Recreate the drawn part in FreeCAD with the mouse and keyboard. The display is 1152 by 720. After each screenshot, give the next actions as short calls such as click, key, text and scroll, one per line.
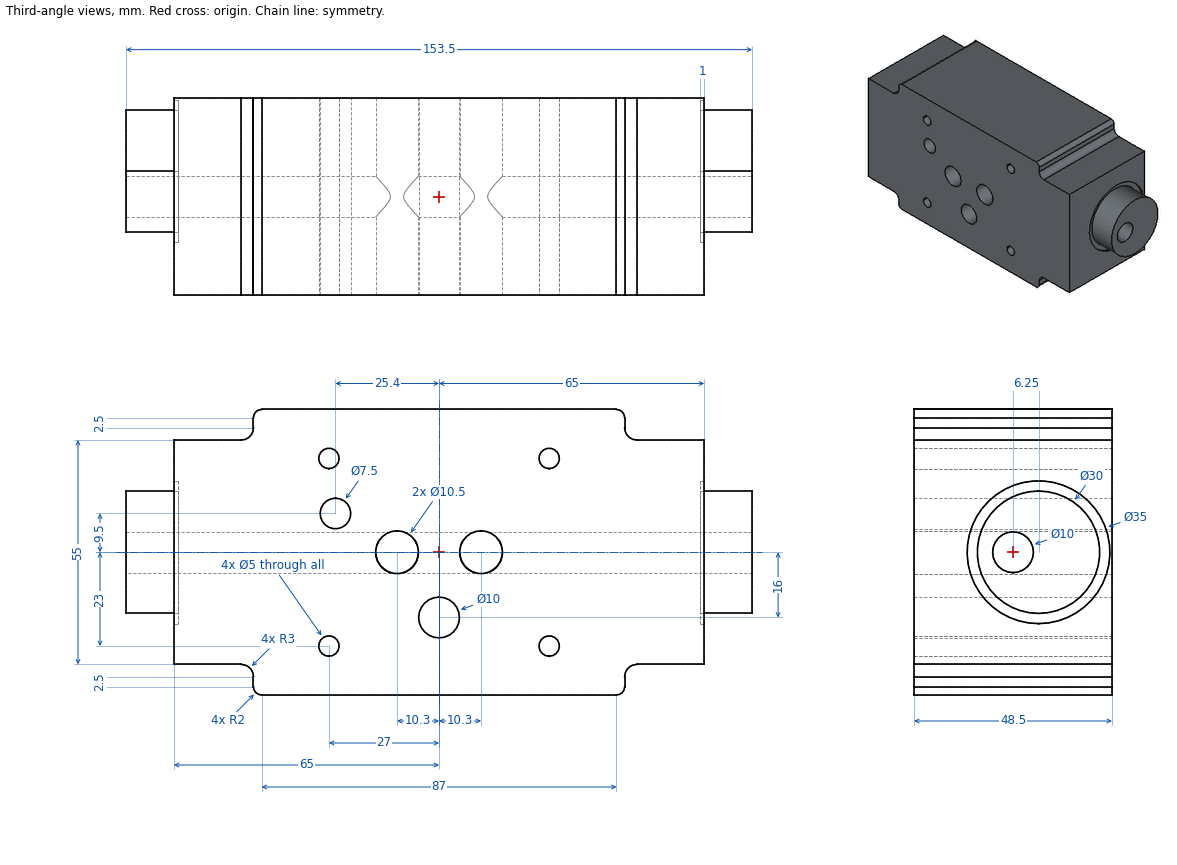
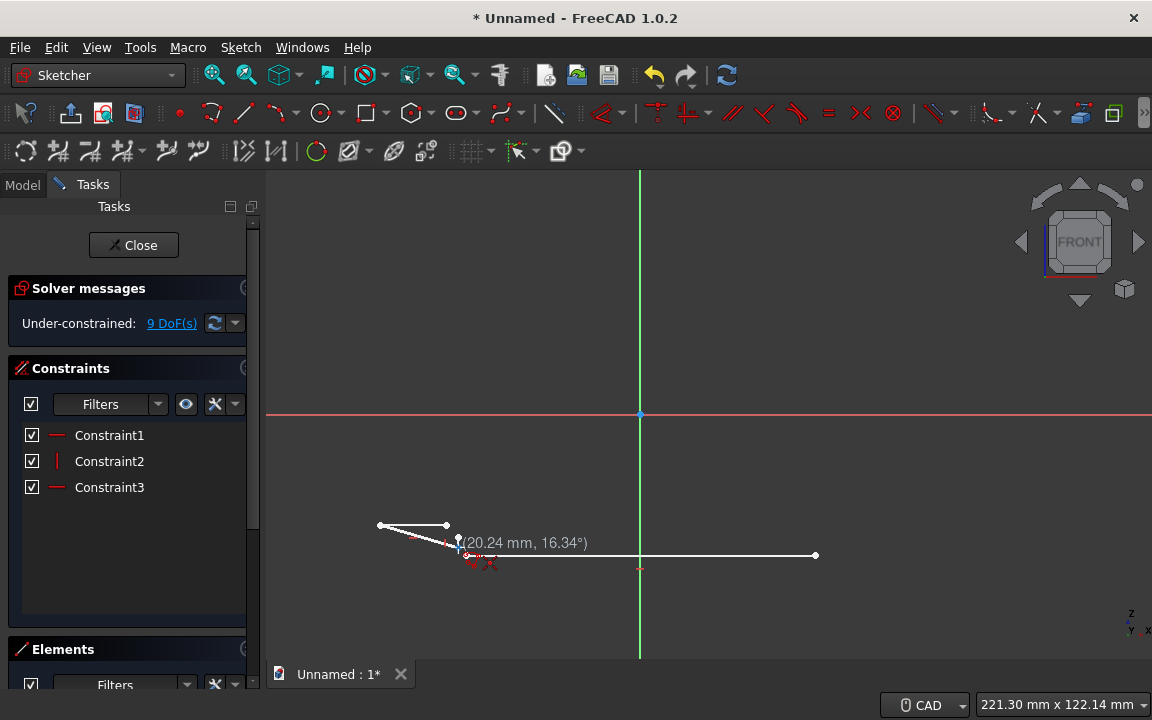
click(380, 305)
click(446, 305)
right_click(446, 305)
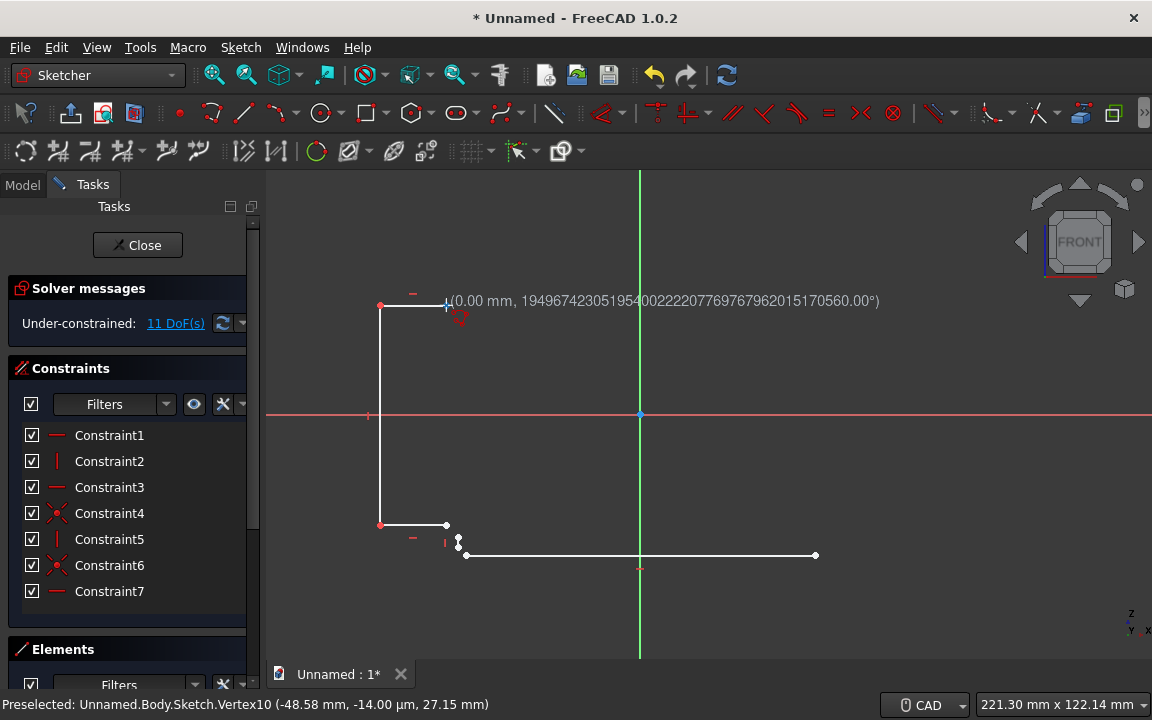
click(244, 114)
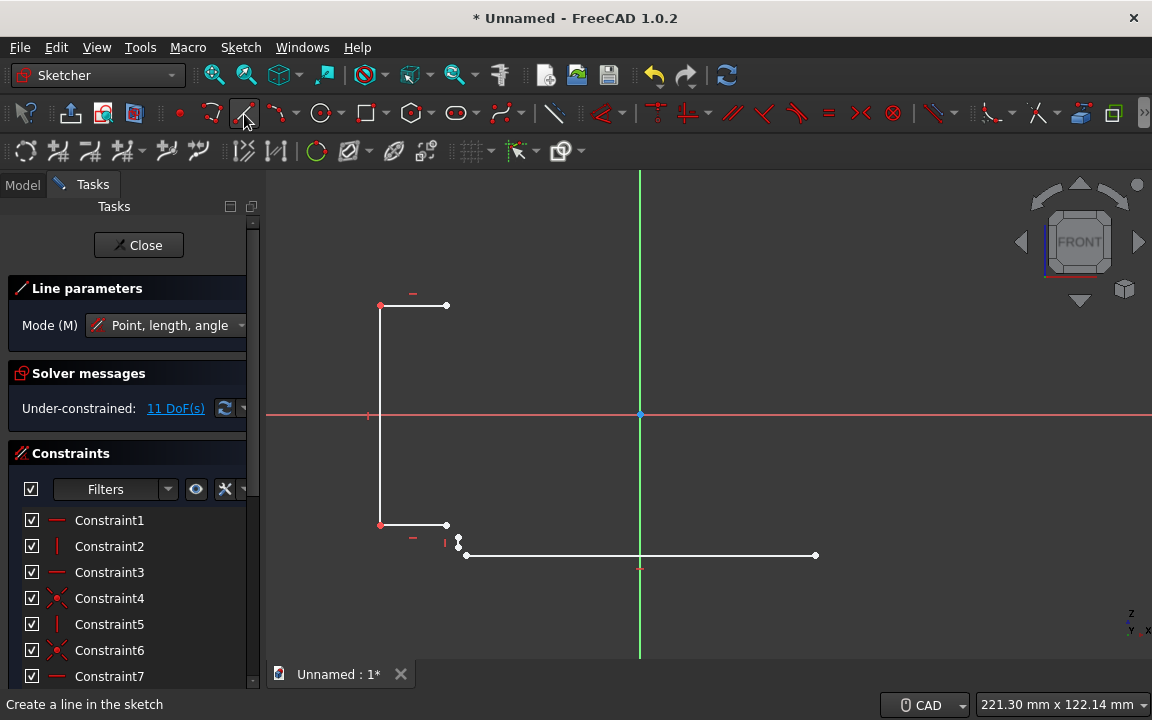
click(458, 293)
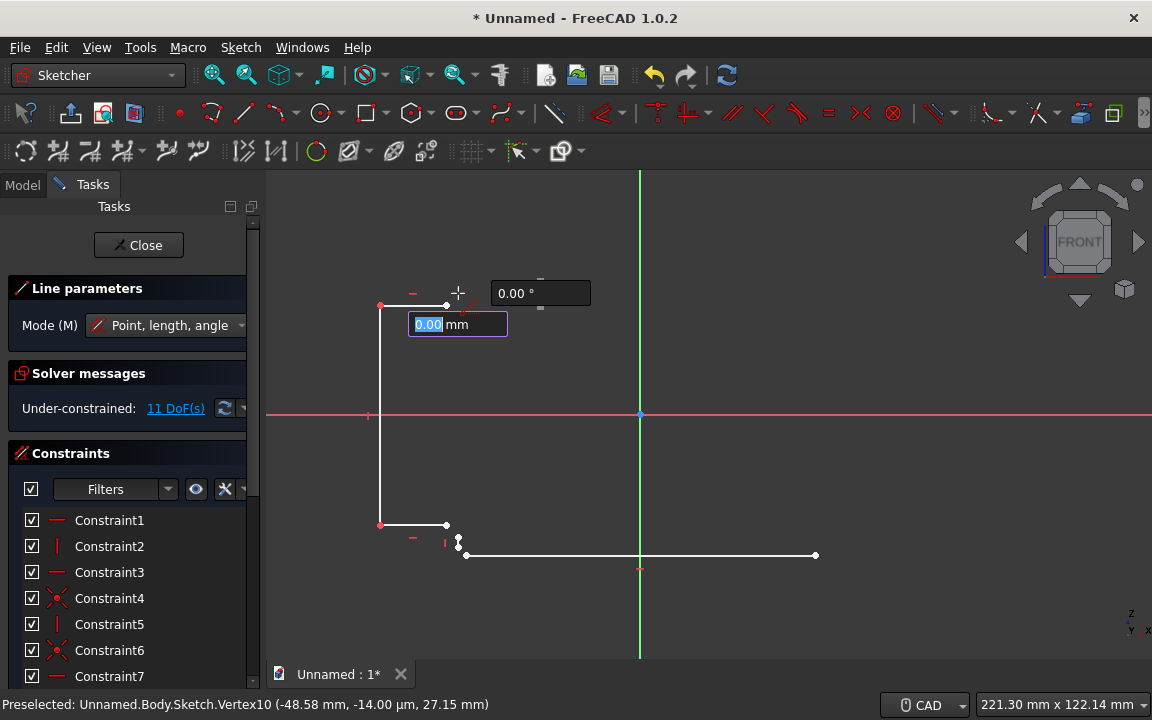
scroll(458, 283, up, 3)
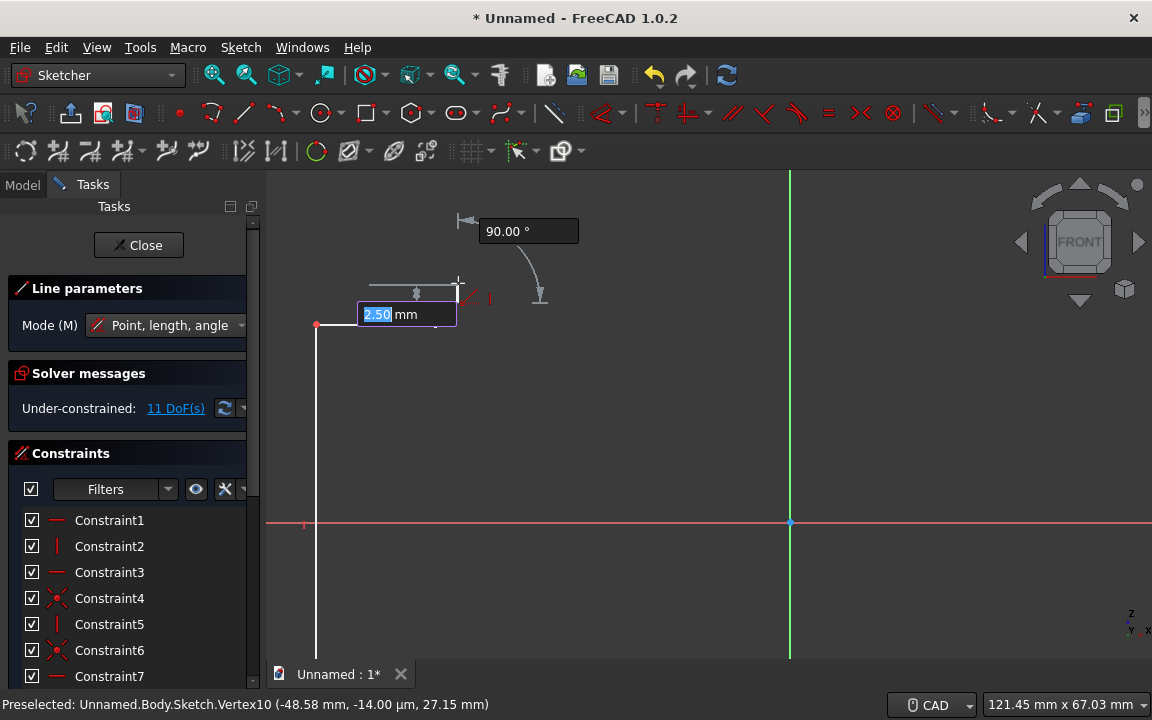
click(458, 282)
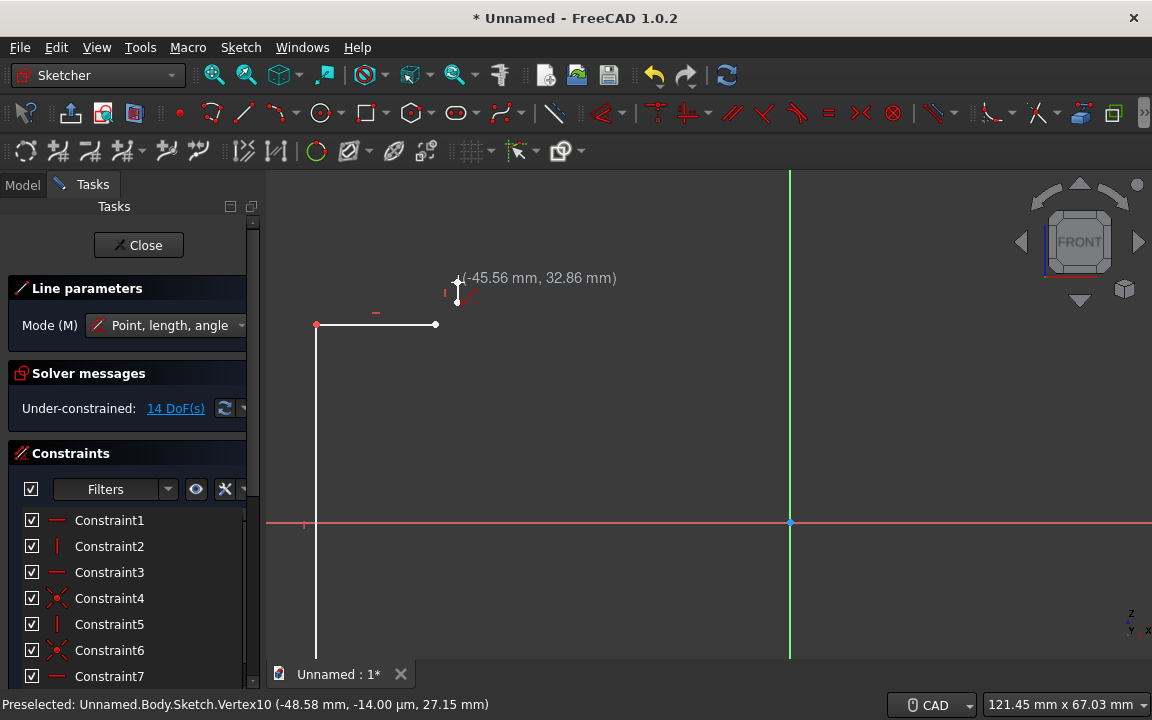
click(473, 267)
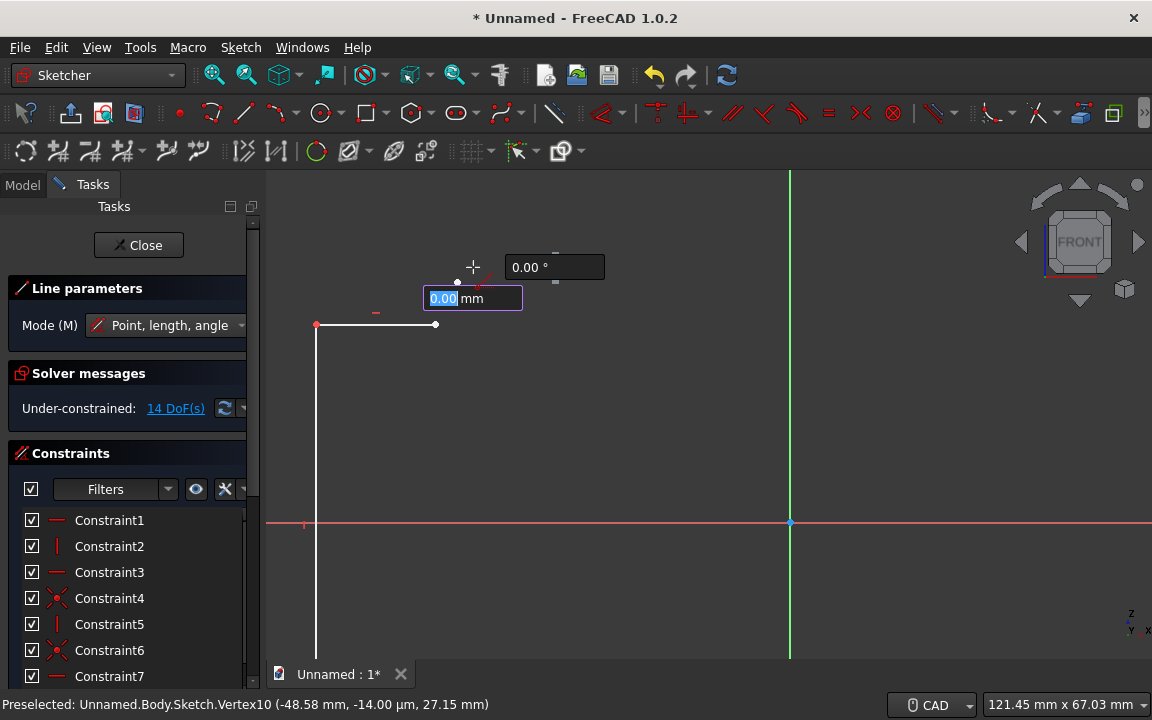
scroll(458, 283, down, 3)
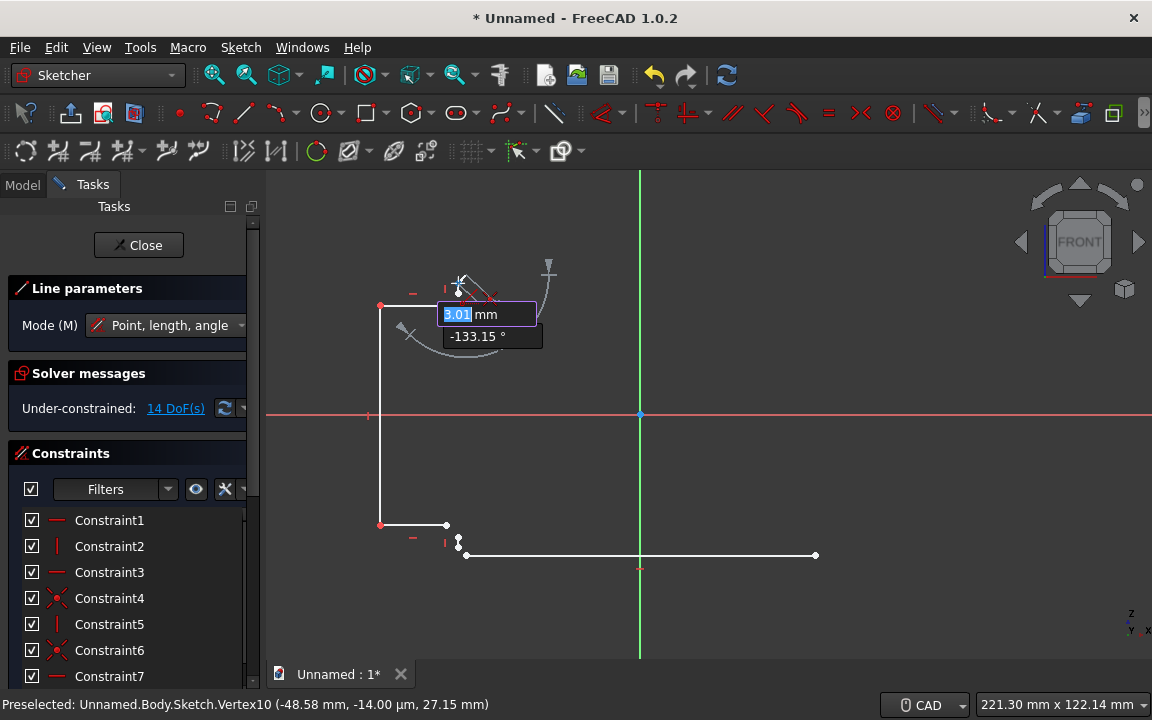
click(815, 274)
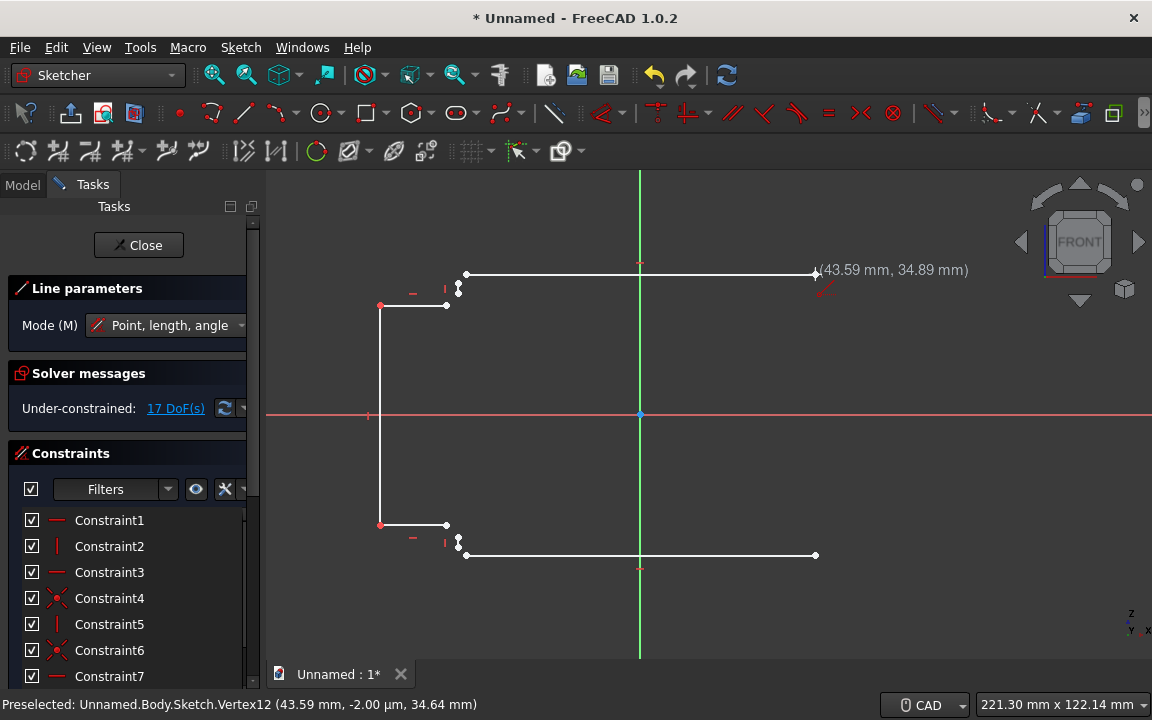
scroll(823, 283, up, 2)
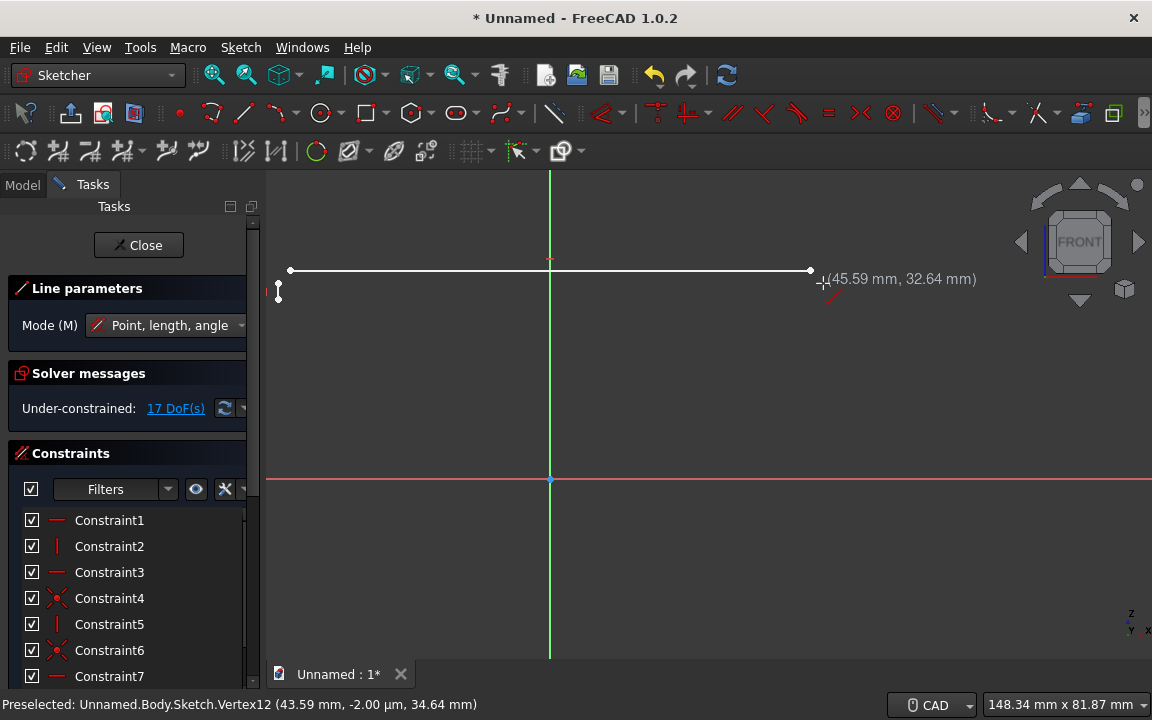
click(822, 282)
click(822, 297)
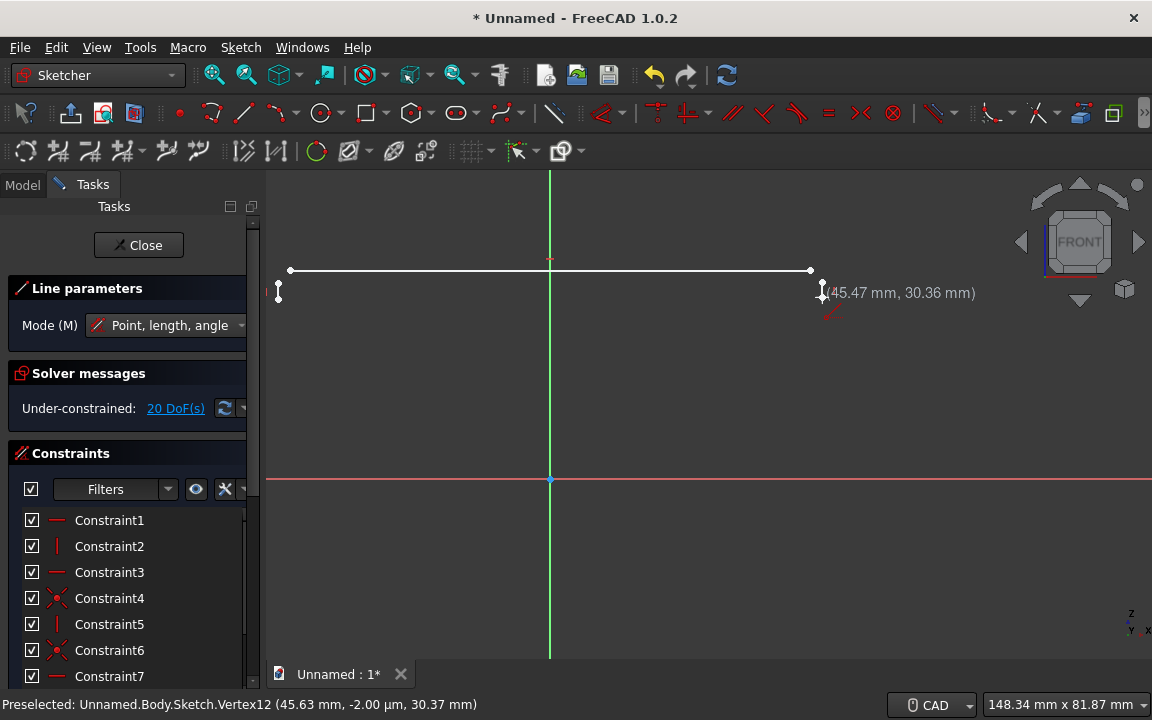
click(212, 114)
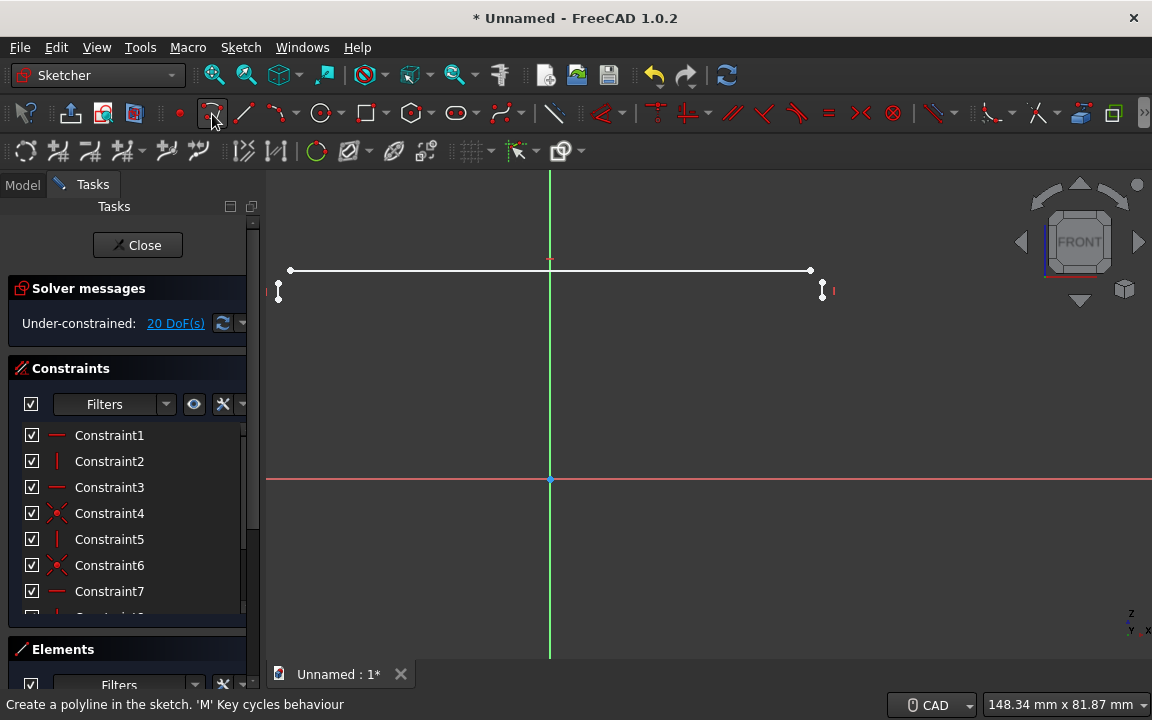
click(840, 315)
click(939, 315)